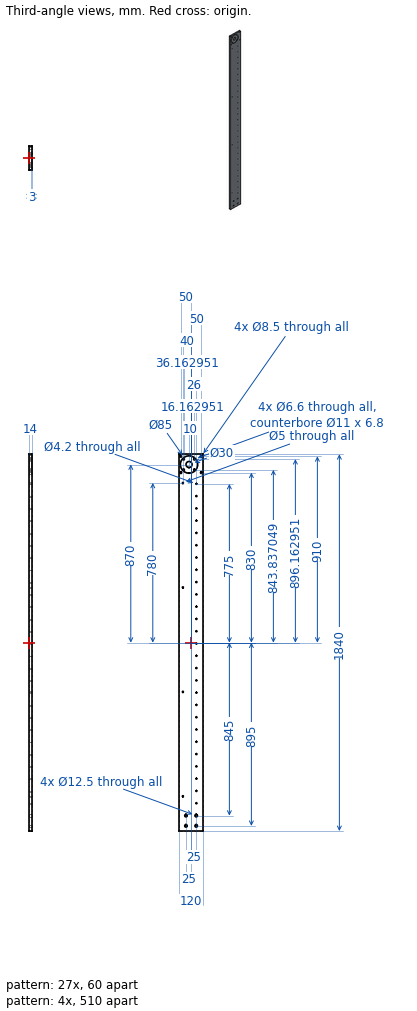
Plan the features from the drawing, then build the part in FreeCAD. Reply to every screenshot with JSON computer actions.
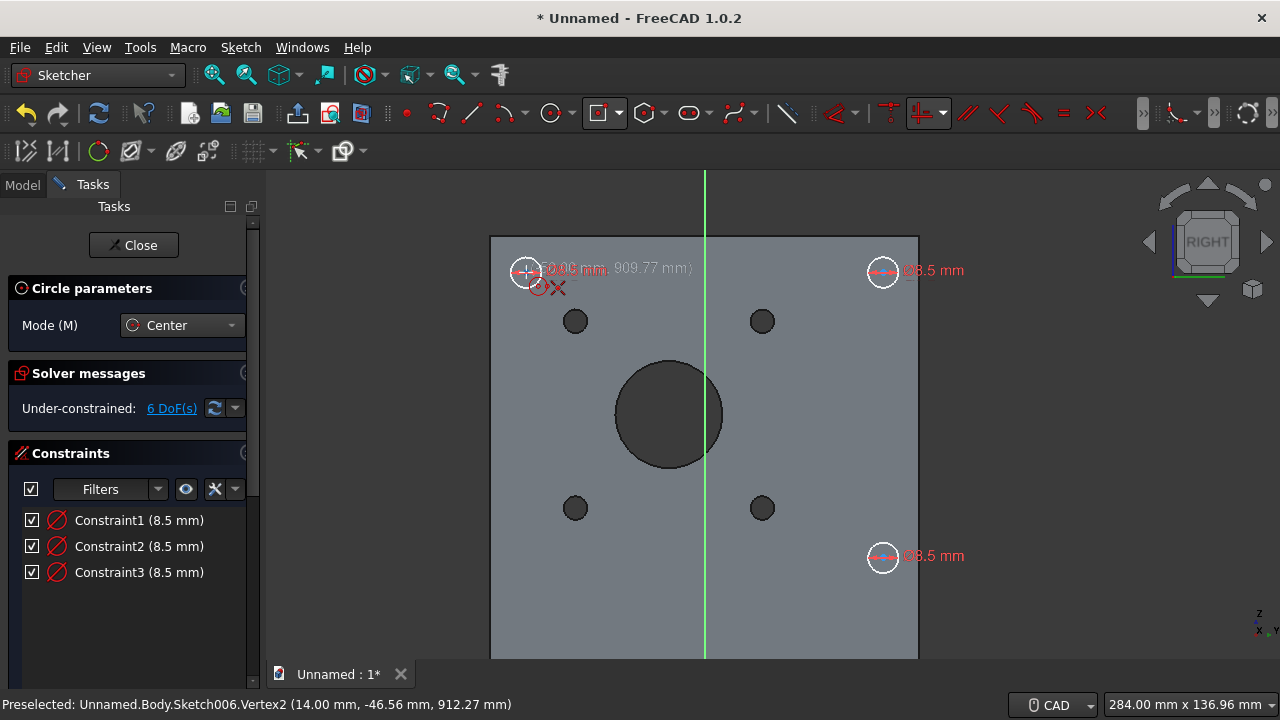
{"action": "scroll", "coordinate": [526, 557], "scroll_direction": "up", "scroll_amount": 3}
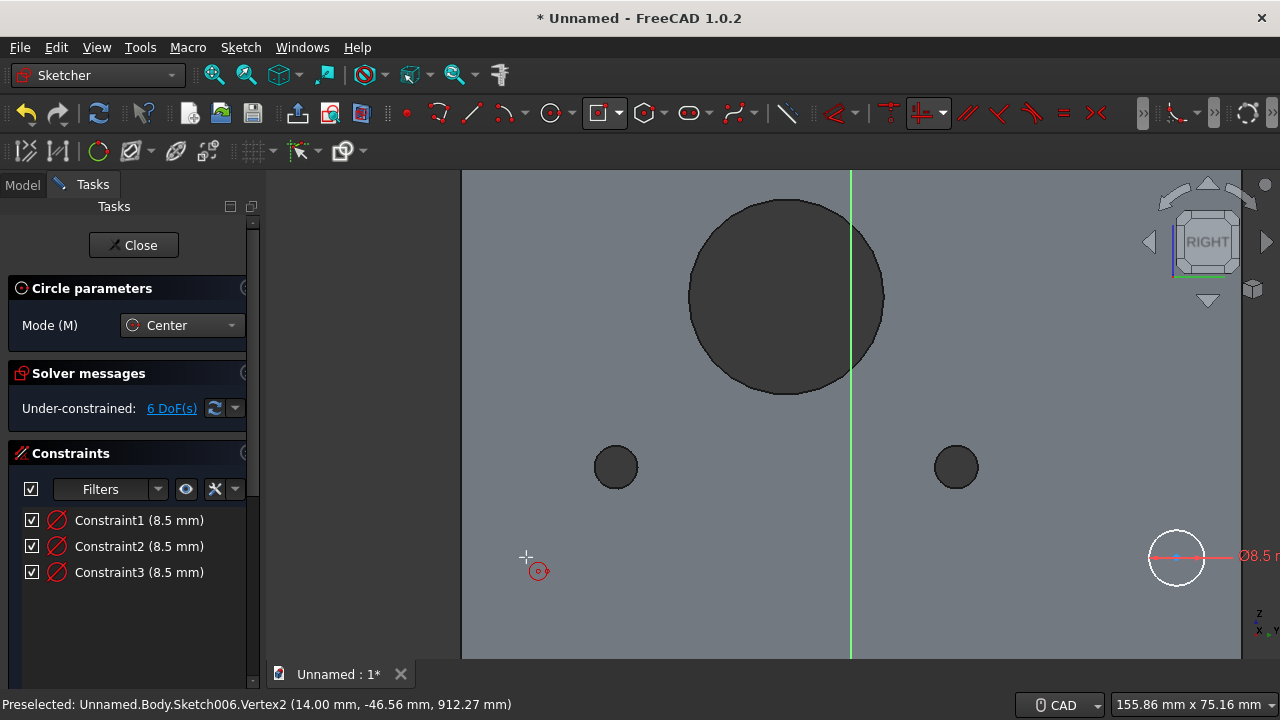
{"action": "left_click", "coordinate": [526, 557]}
{"action": "mouse_move", "coordinate": [546, 538]}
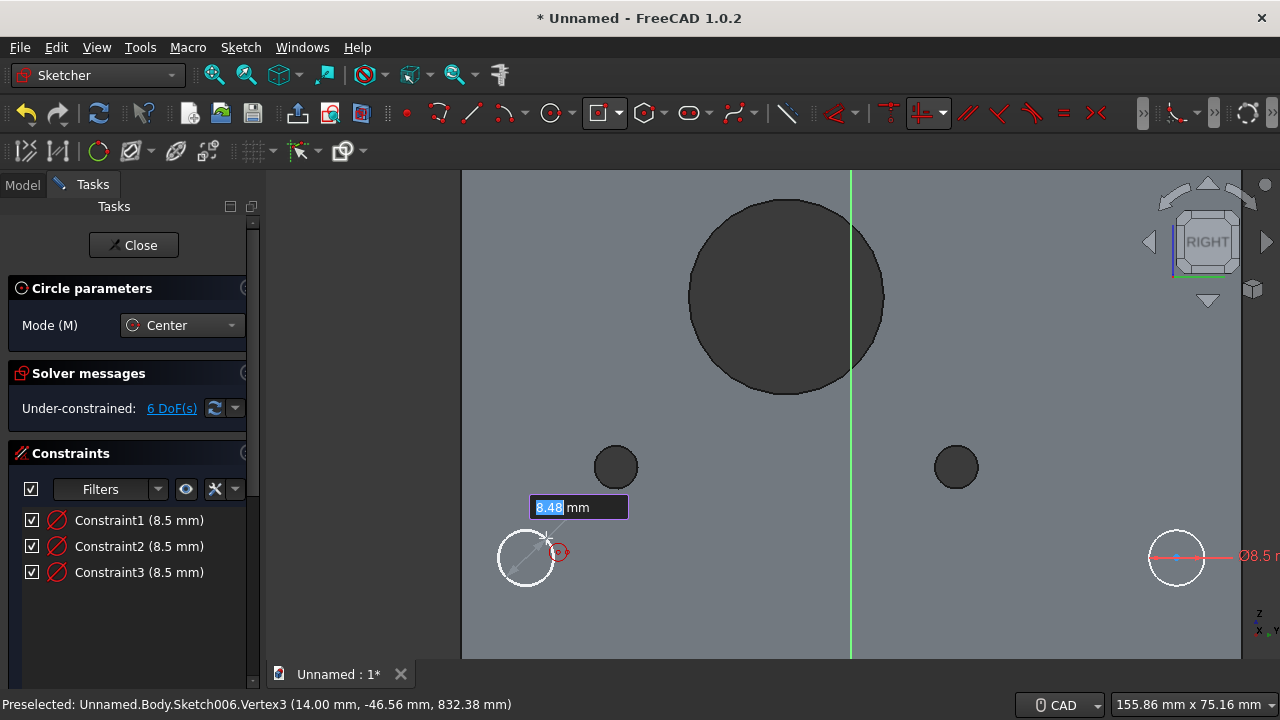
{"action": "type", "text": "8.5"}
{"action": "key", "text": "Return"}
{"action": "key", "text": "Escape"}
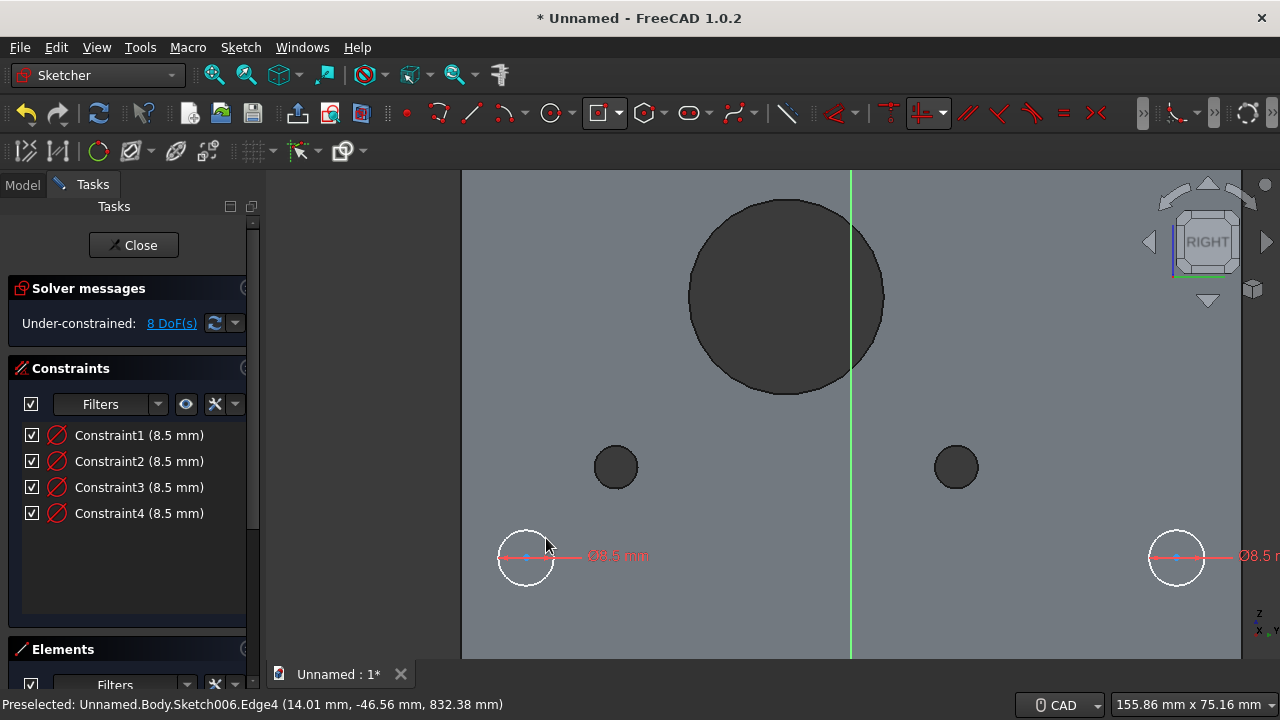
{"action": "scroll", "coordinate": [526, 557], "scroll_direction": "down", "scroll_amount": 3}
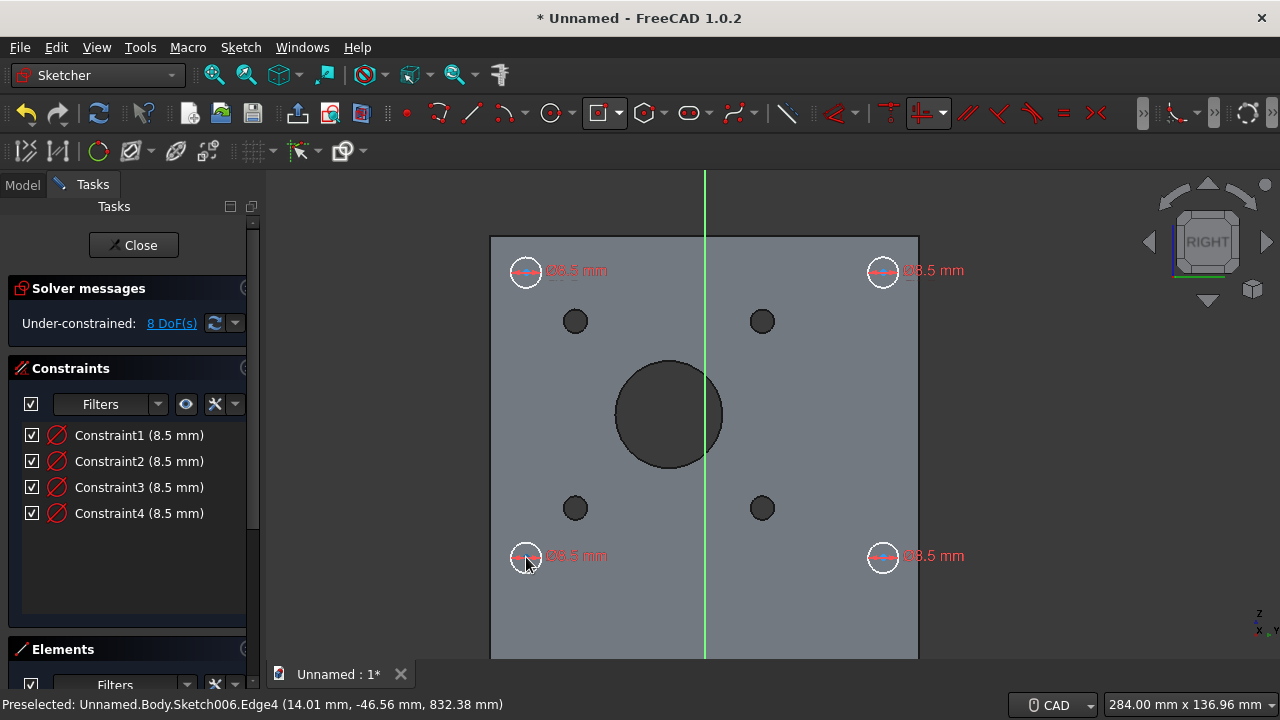
{"action": "left_click", "coordinate": [883, 273]}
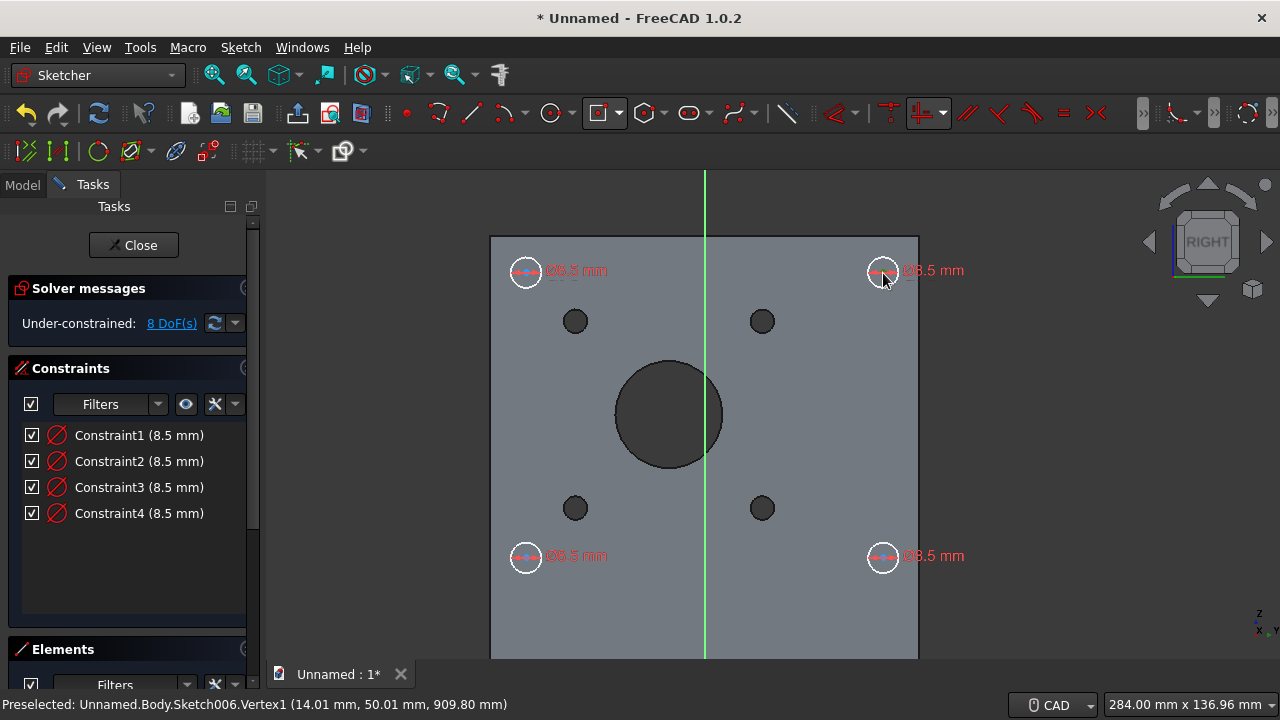
{"action": "left_click", "coordinate": [883, 558]}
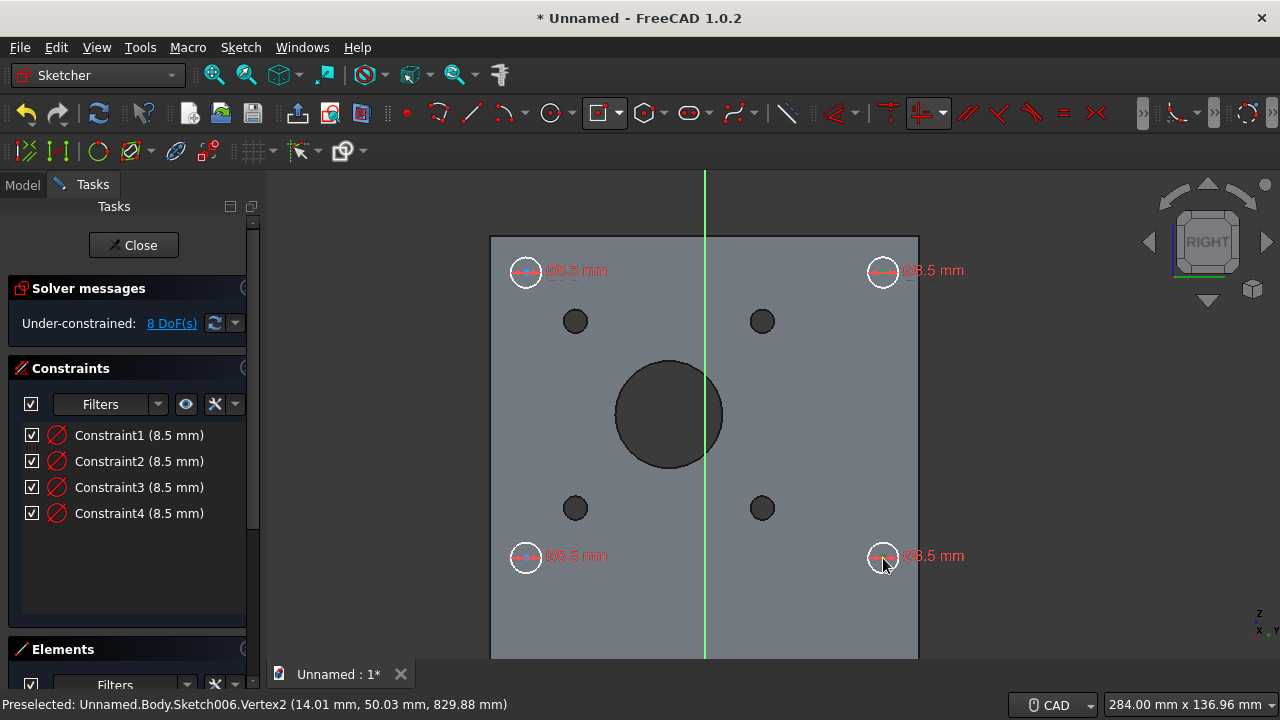
{"action": "left_click", "coordinate": [946, 114]}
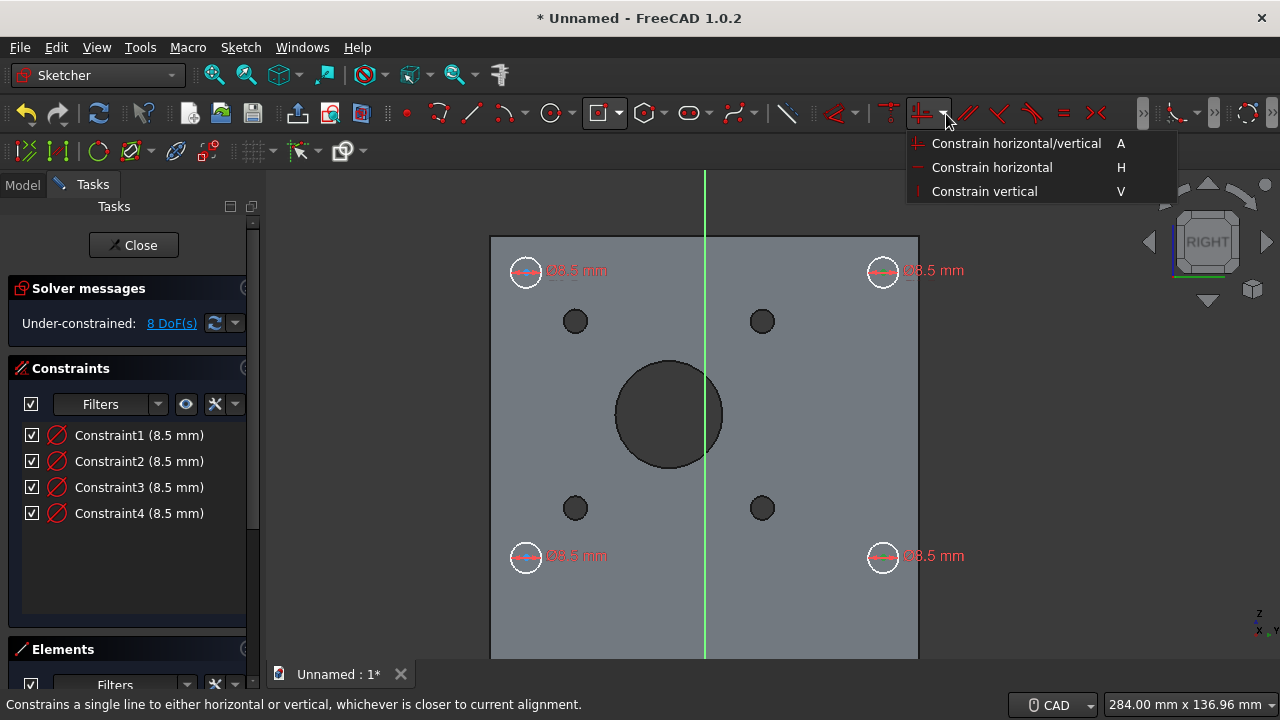
{"action": "left_click", "coordinate": [1042, 191]}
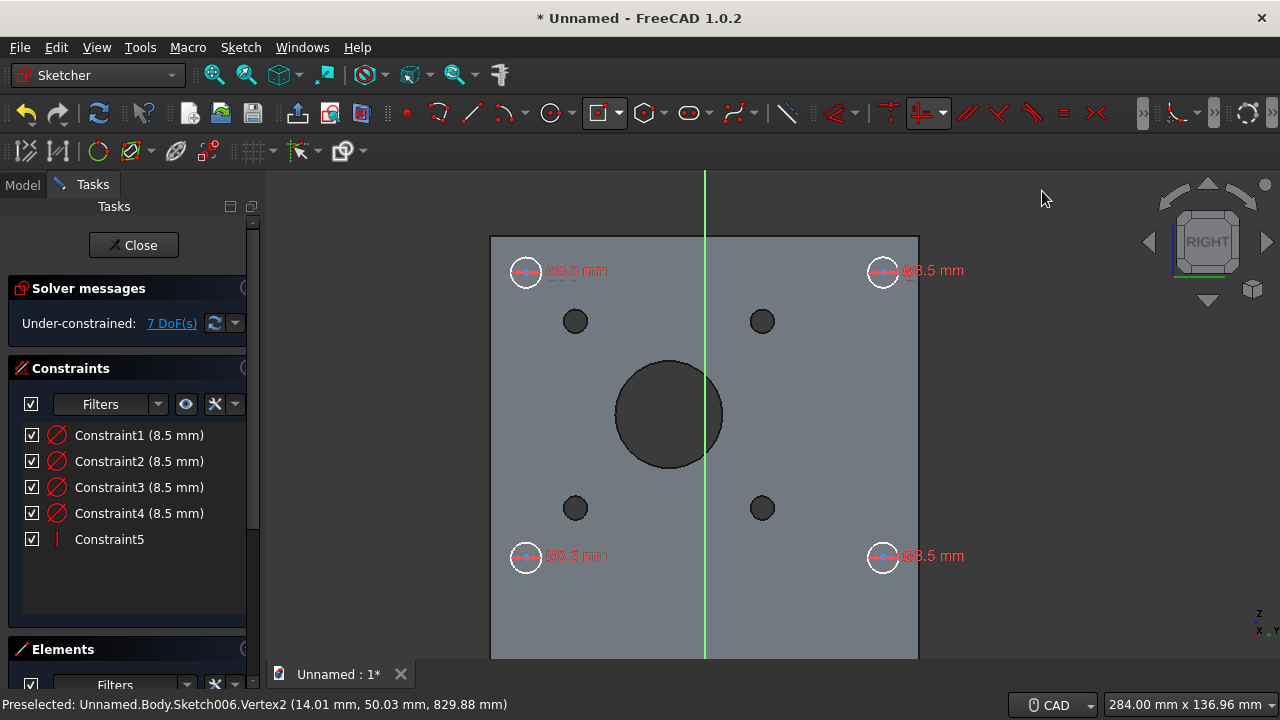
{"action": "left_click", "coordinate": [883, 273]}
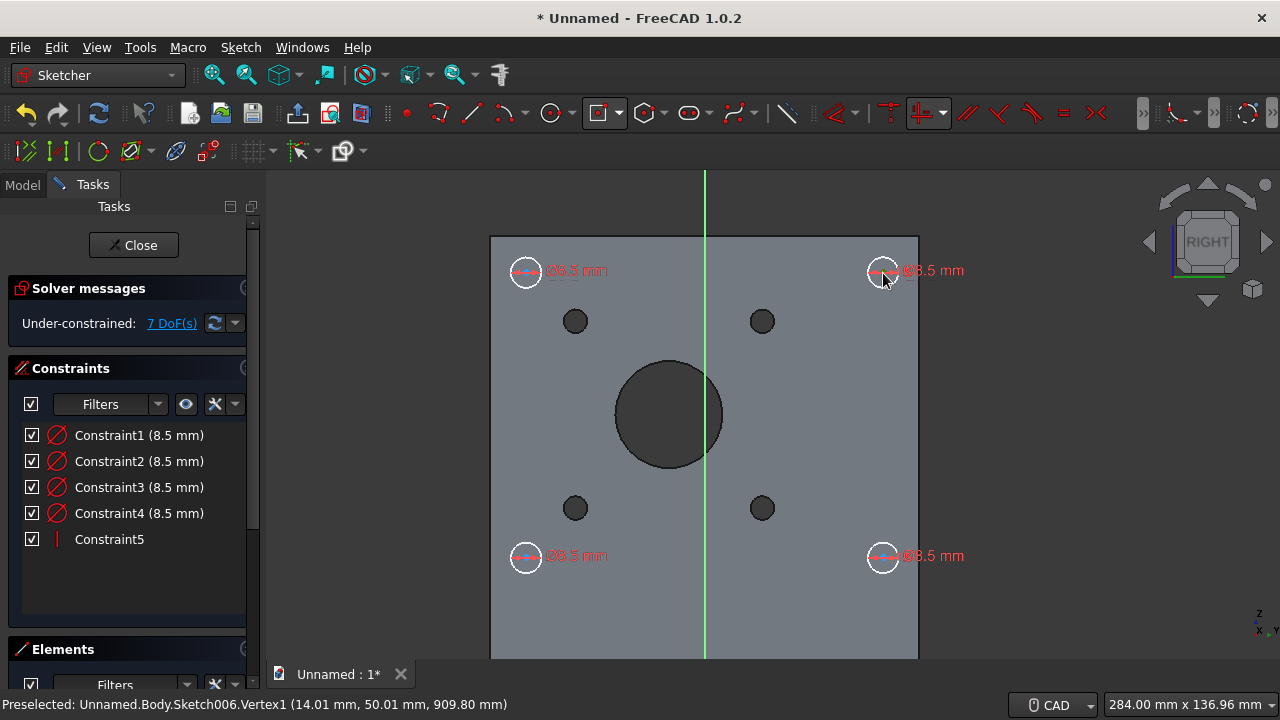
{"action": "left_click", "coordinate": [526, 273]}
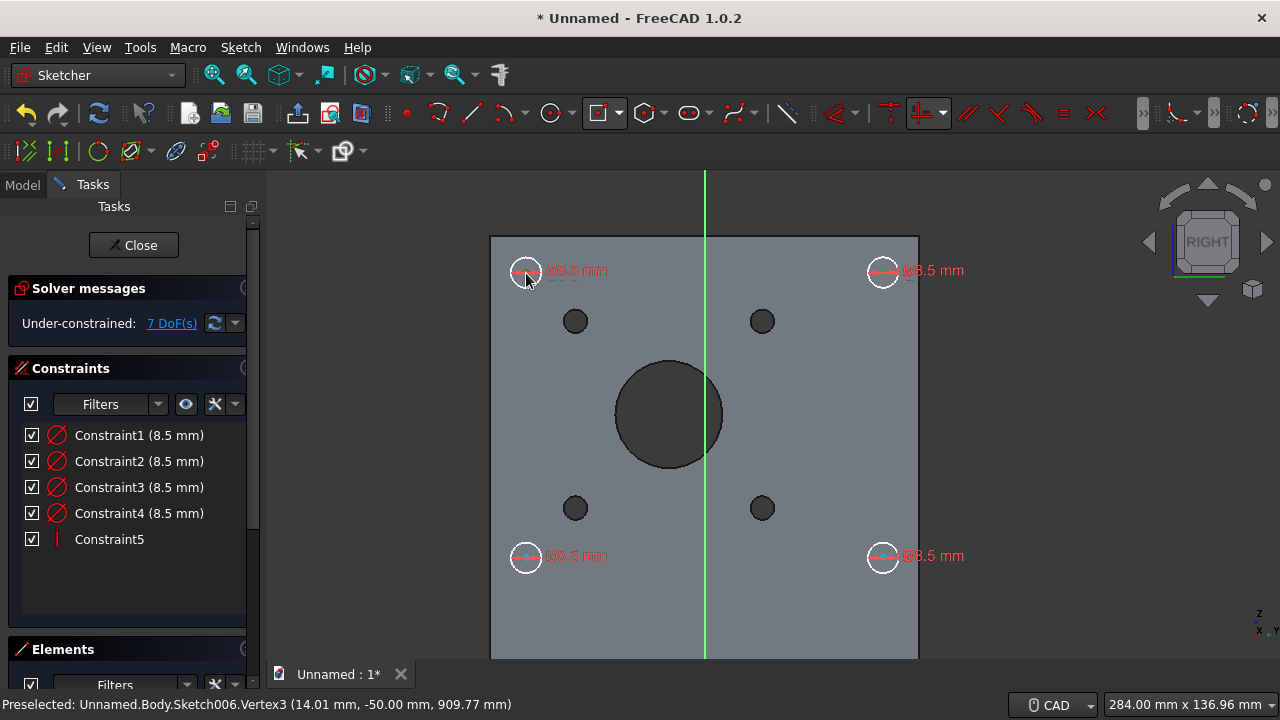
{"action": "key", "text": "h"}